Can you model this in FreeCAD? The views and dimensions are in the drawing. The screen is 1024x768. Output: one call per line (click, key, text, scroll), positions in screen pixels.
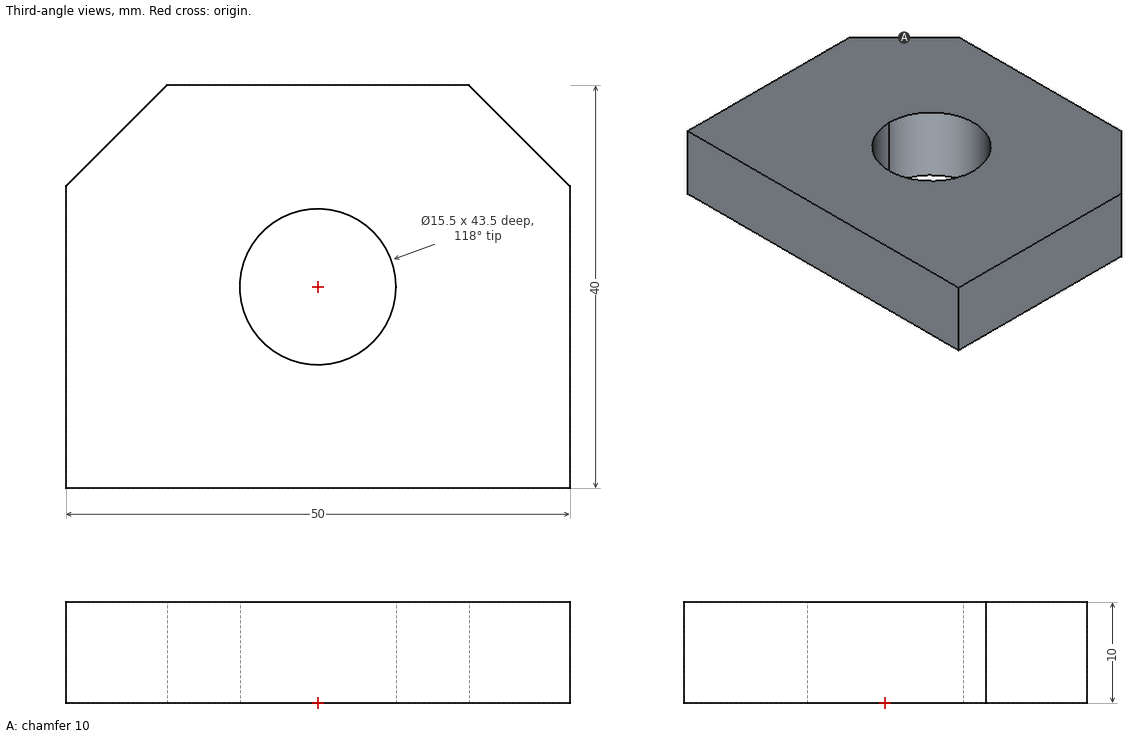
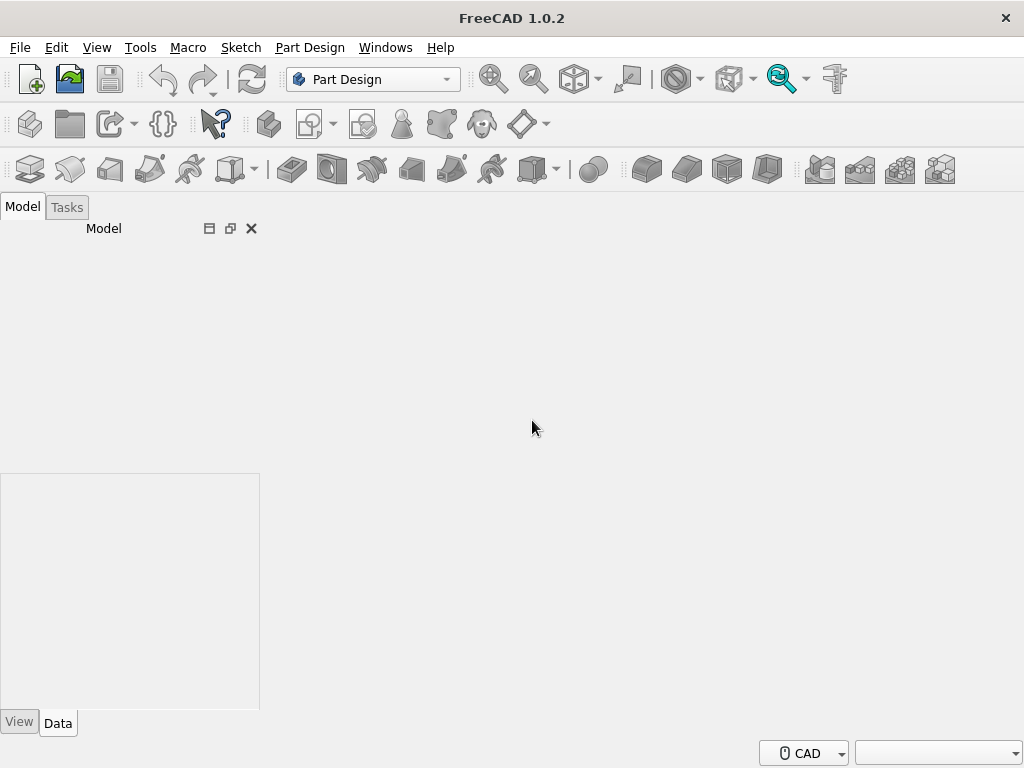
key(ctrl+n)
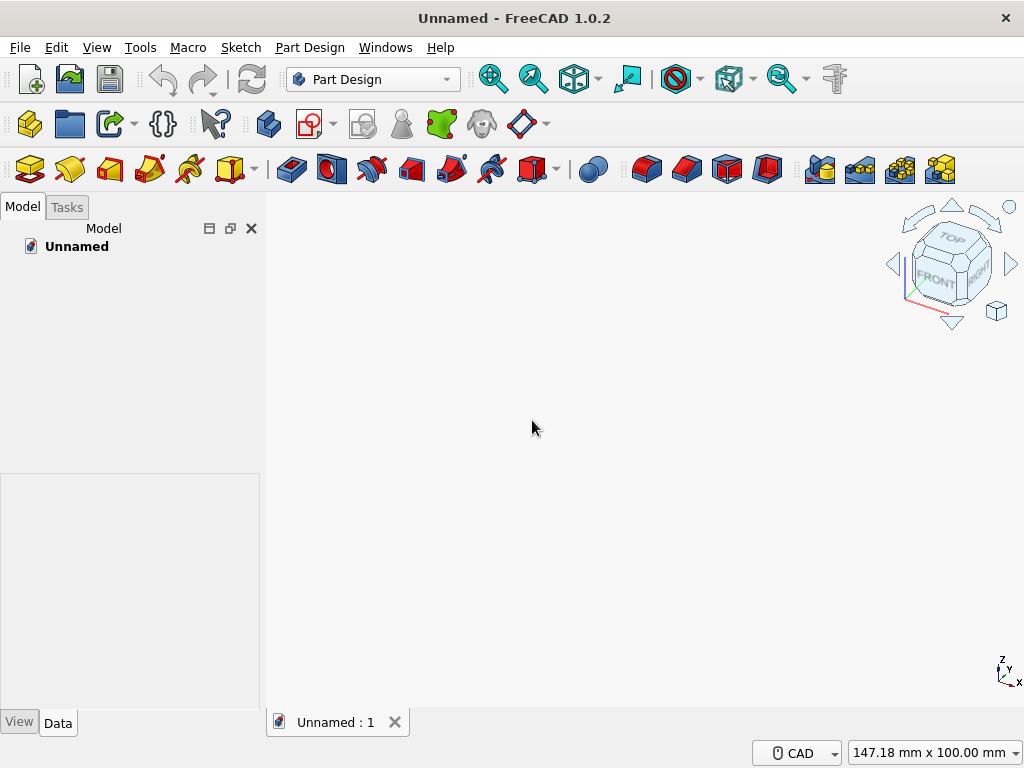
click(310, 124)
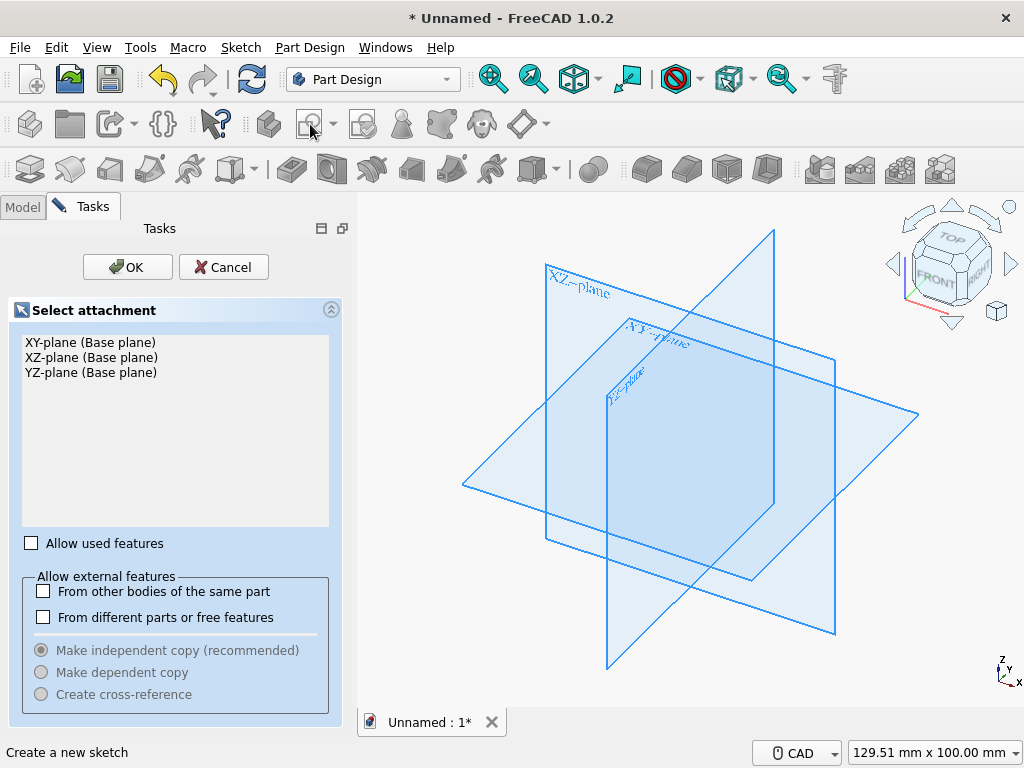
click(82, 342)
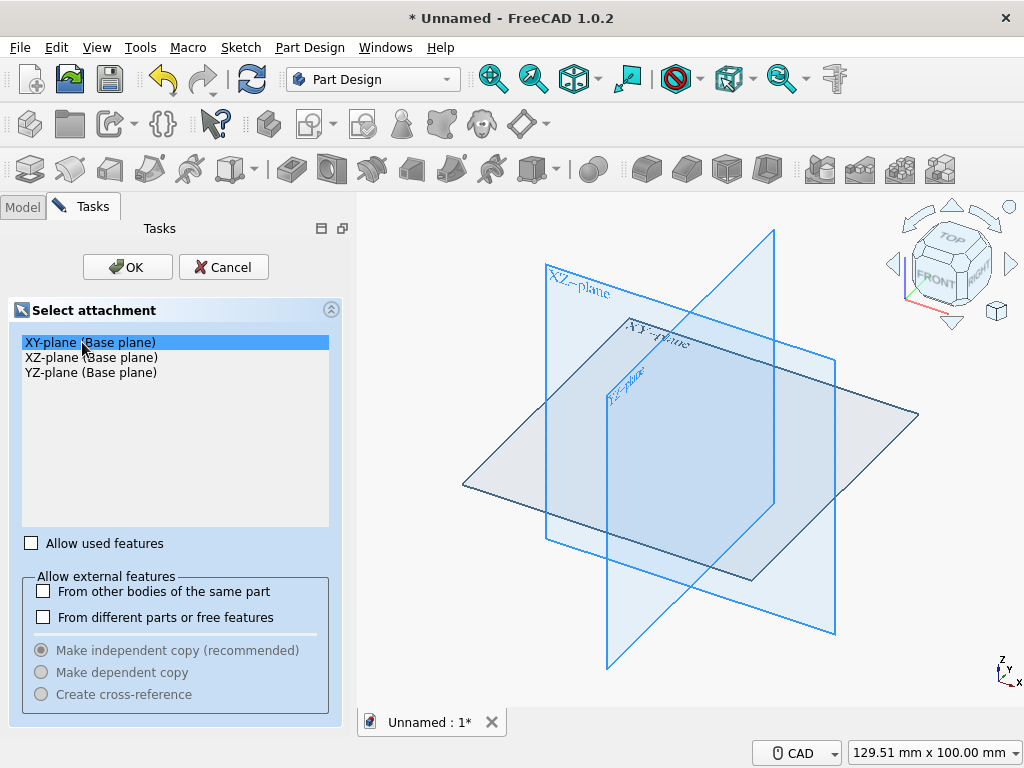
click(128, 267)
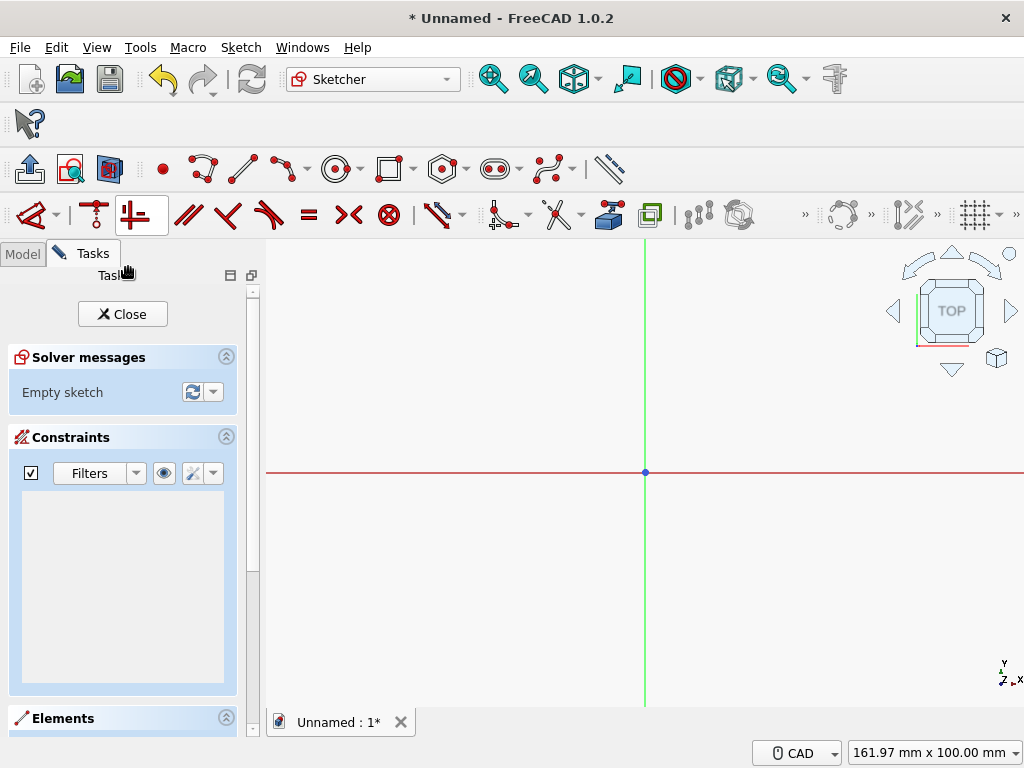
scroll(784, 473, up, 2)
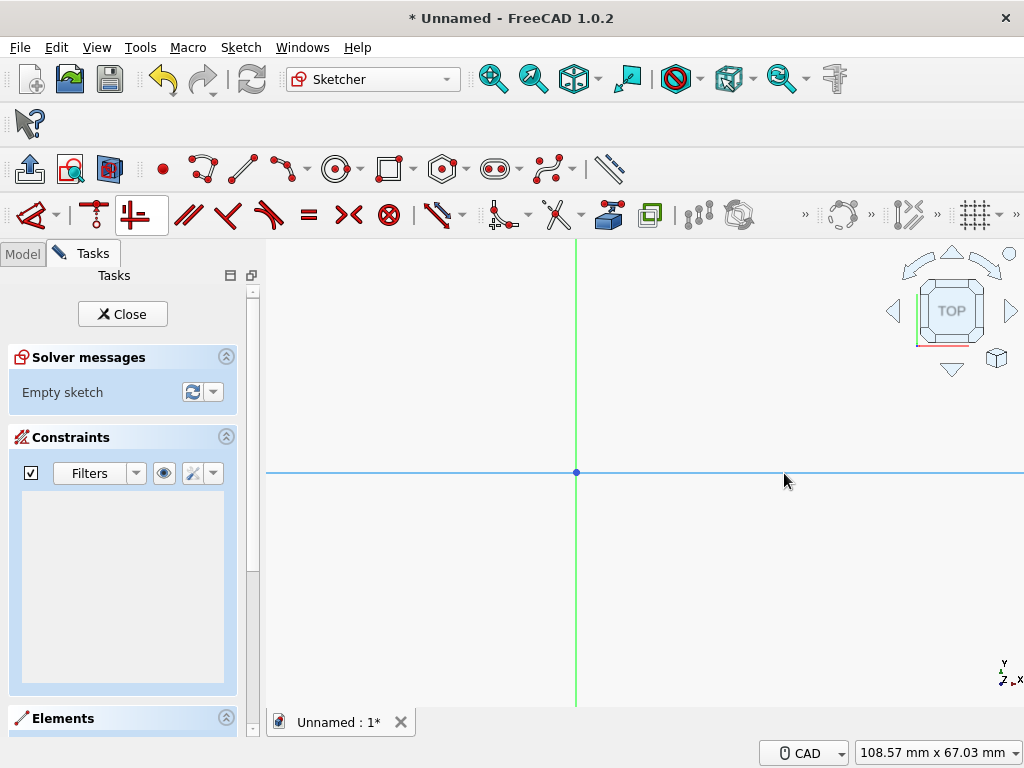
key(g)
key(v)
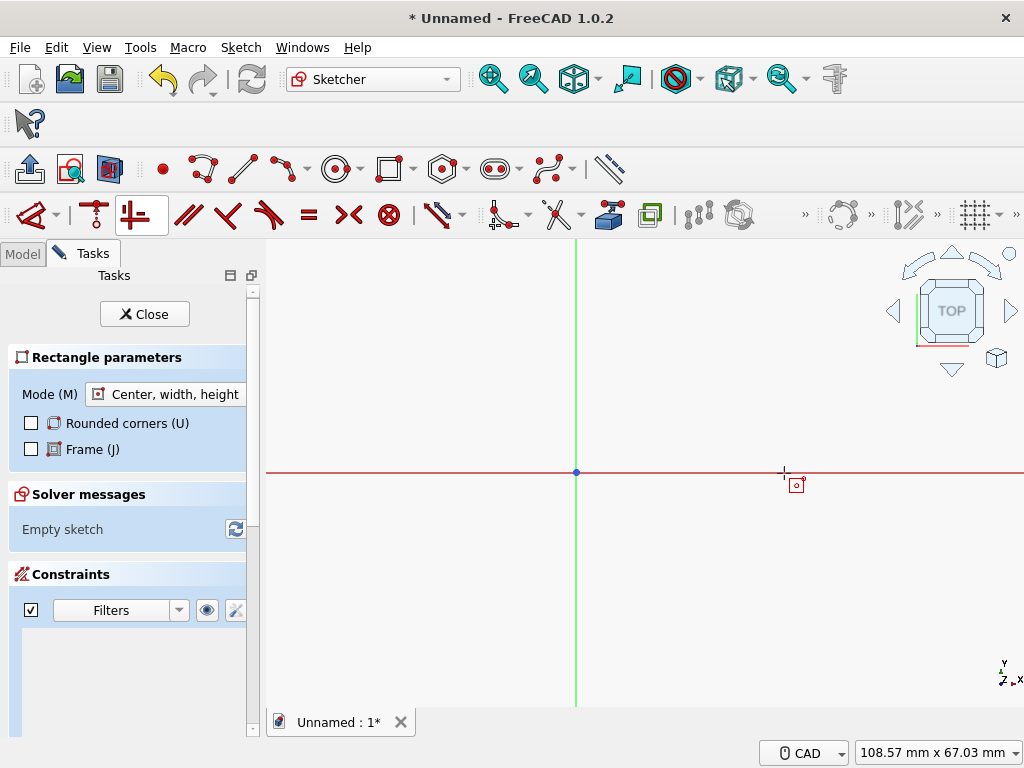
click(576, 473)
click(751, 333)
key(Escape)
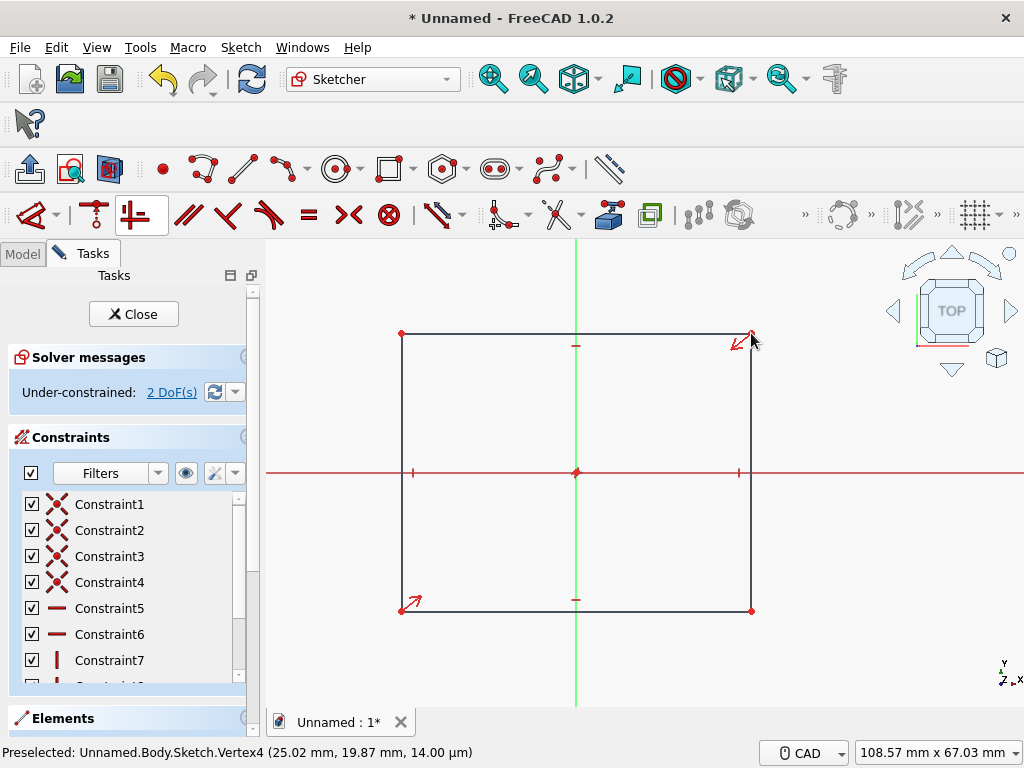
click(32, 216)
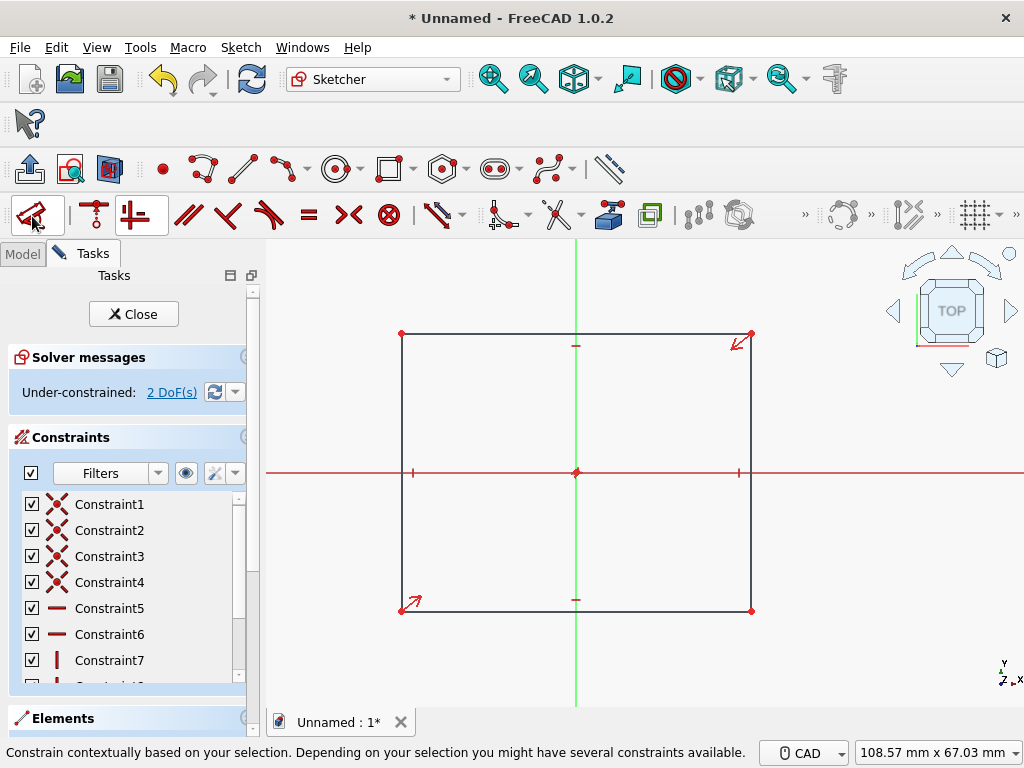
click(506, 612)
click(496, 646)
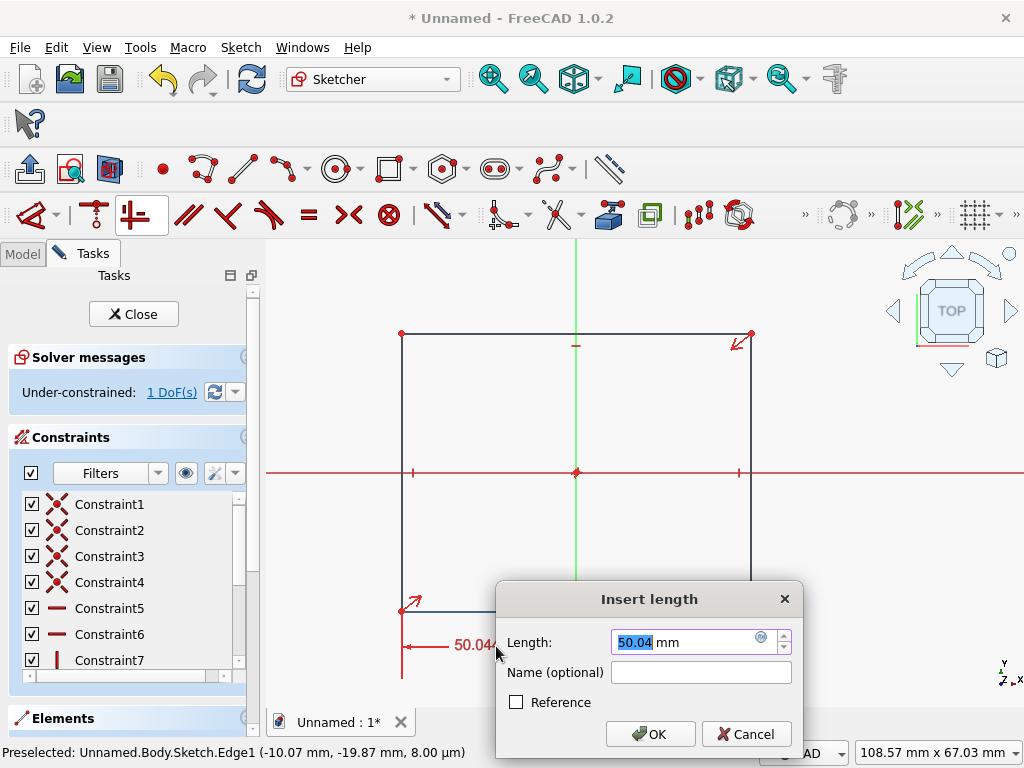
text(50)
key(Return)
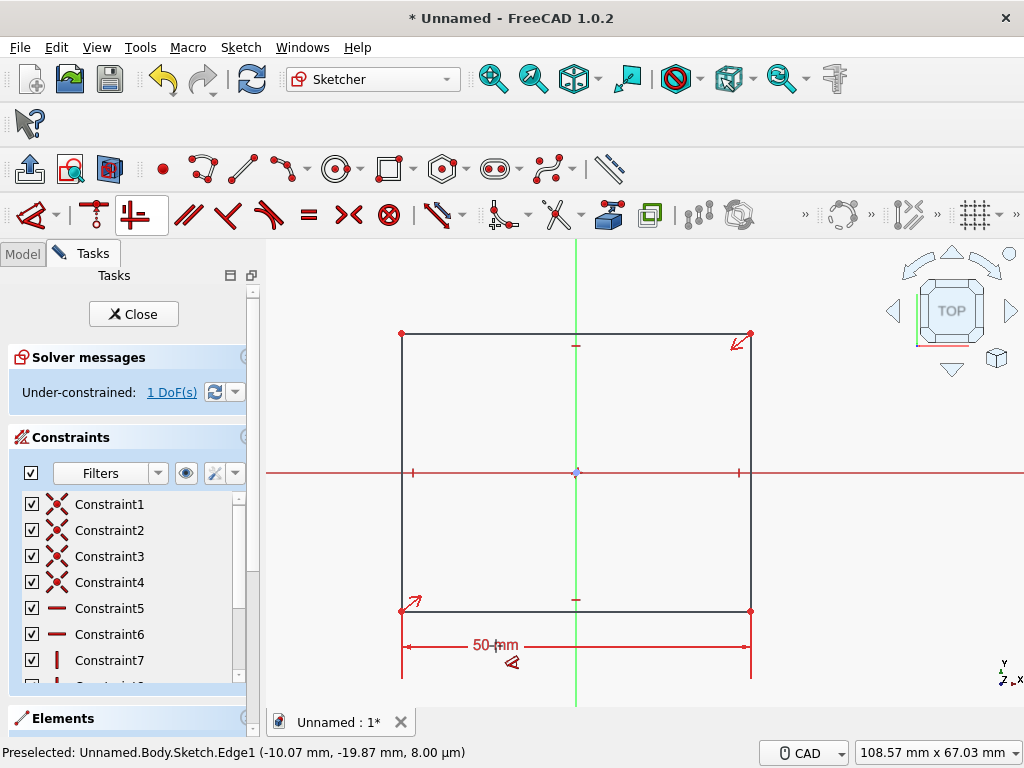
click(751, 528)
click(785, 409)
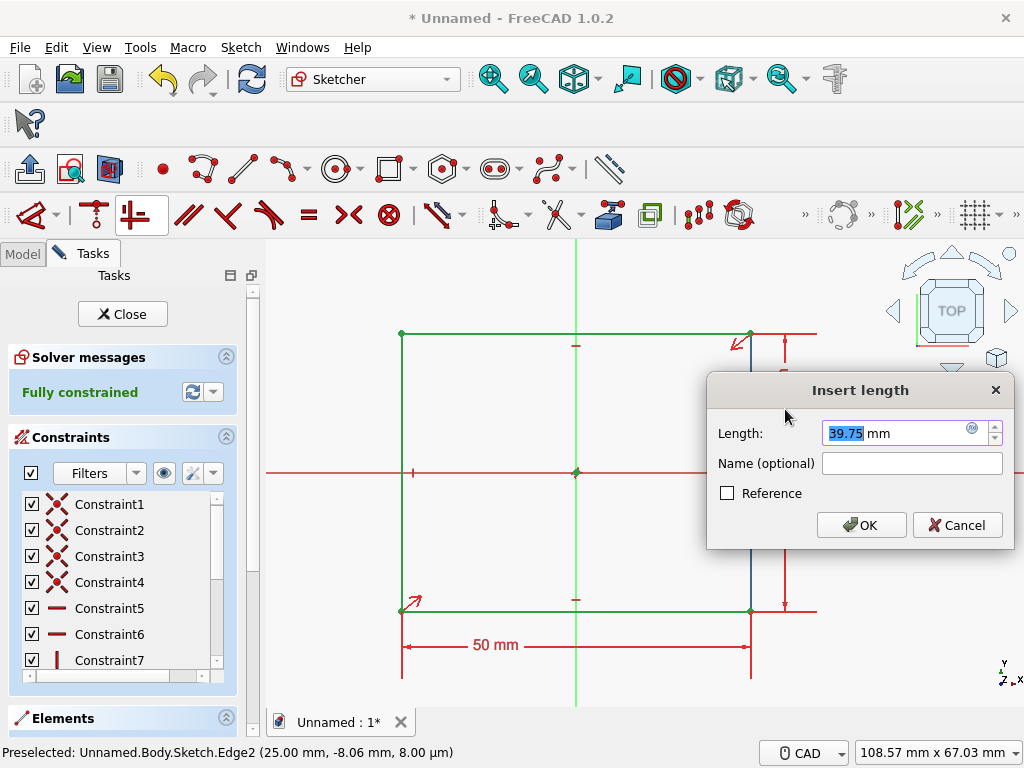
text(40)
key(Return)
key(Escape)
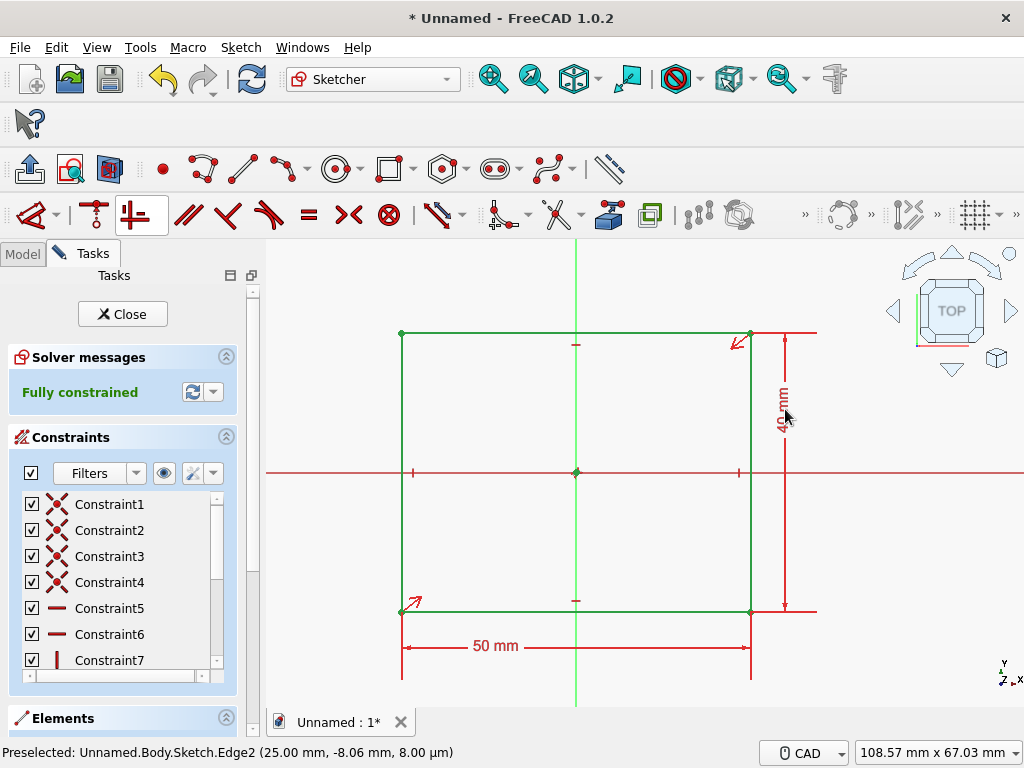
click(123, 314)